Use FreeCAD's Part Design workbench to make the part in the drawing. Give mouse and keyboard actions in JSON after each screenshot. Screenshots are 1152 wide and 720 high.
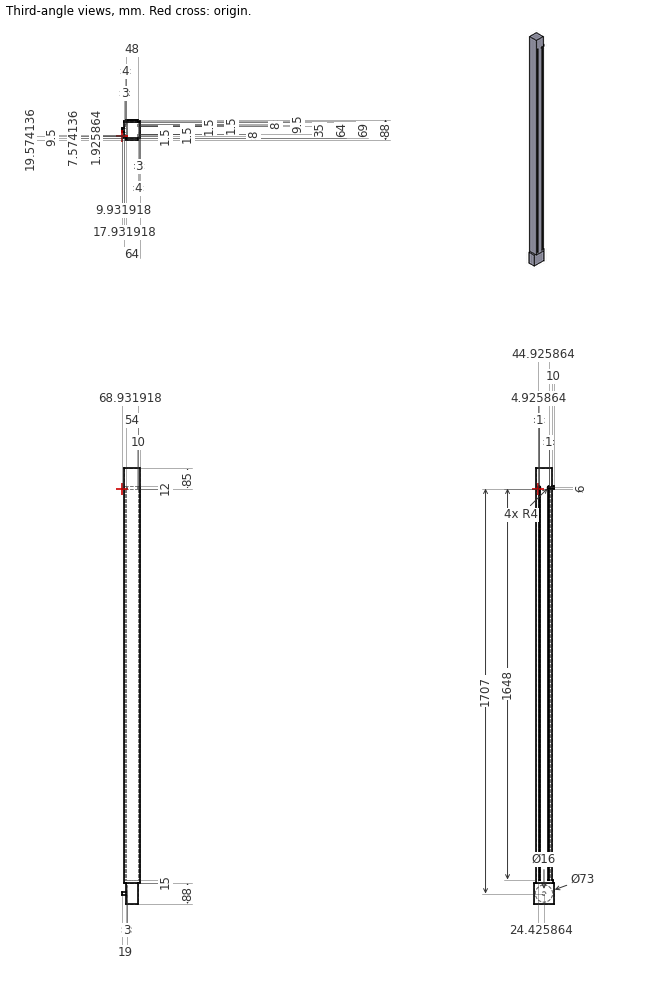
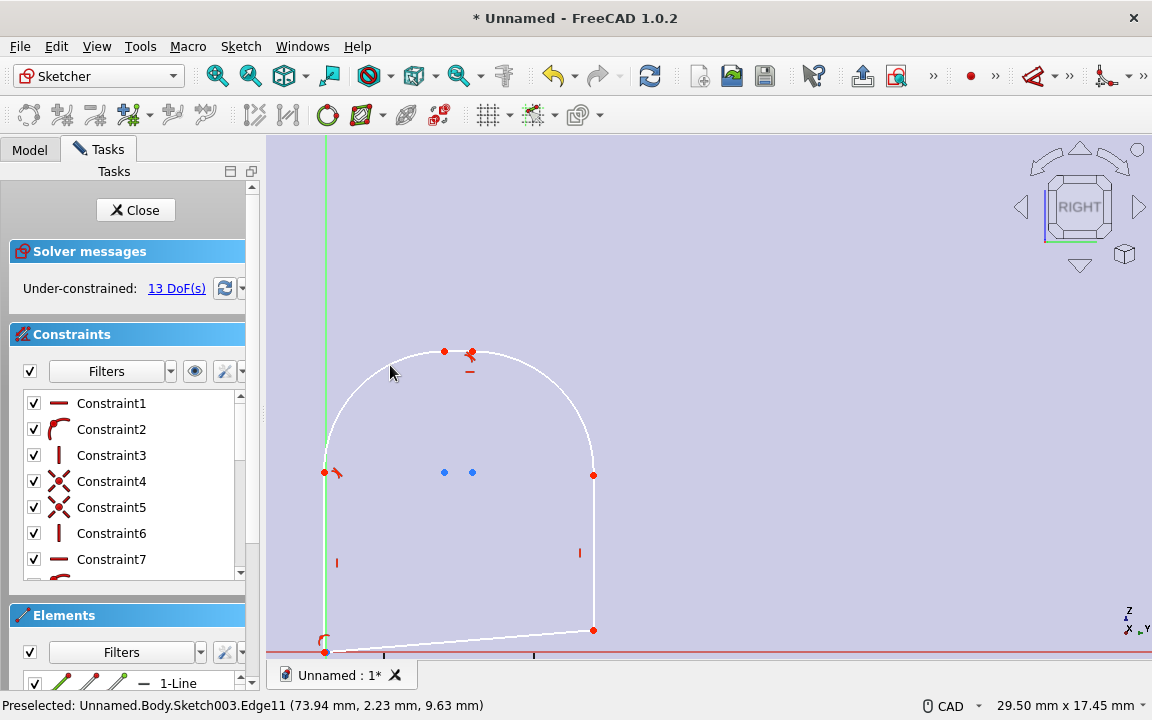
{"action": "left_click", "coordinate": [594, 584]}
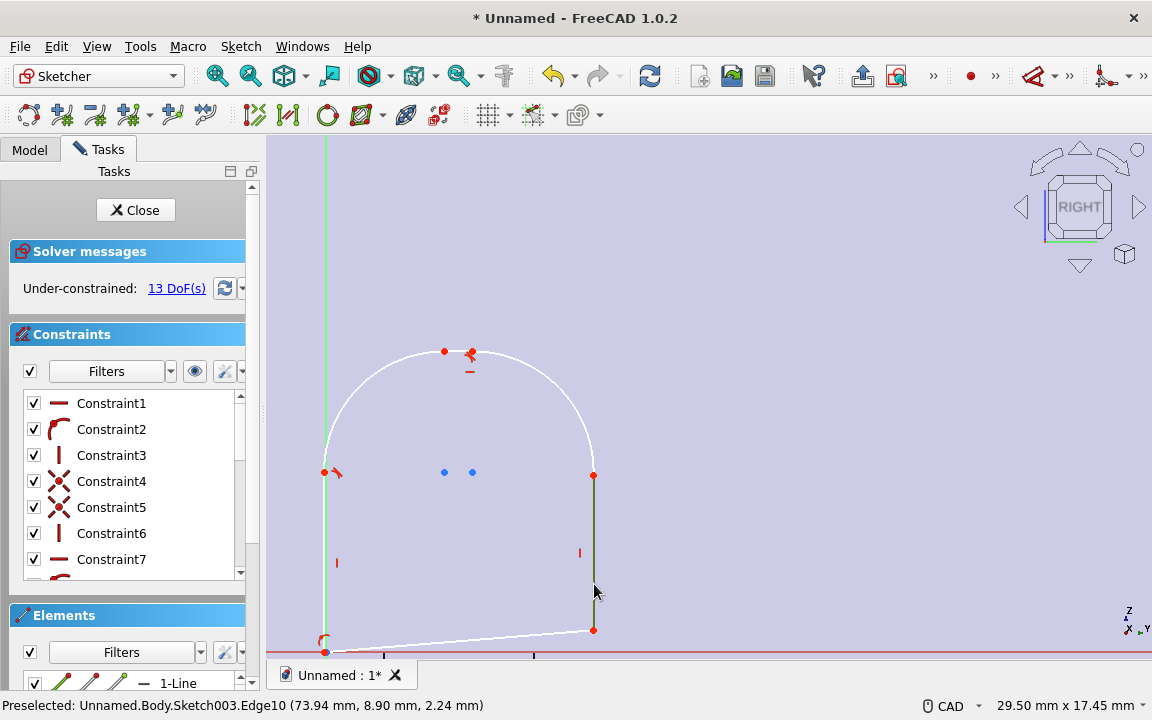
{"action": "left_click", "coordinate": [581, 419]}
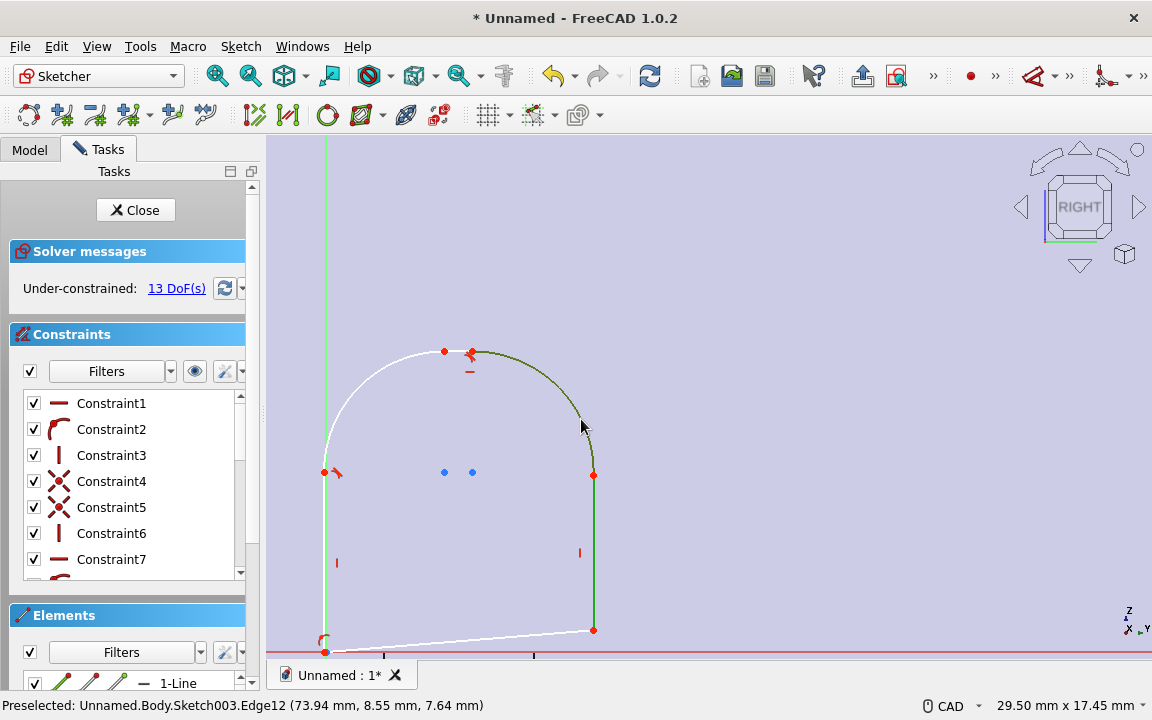
{"action": "key", "text": "t"}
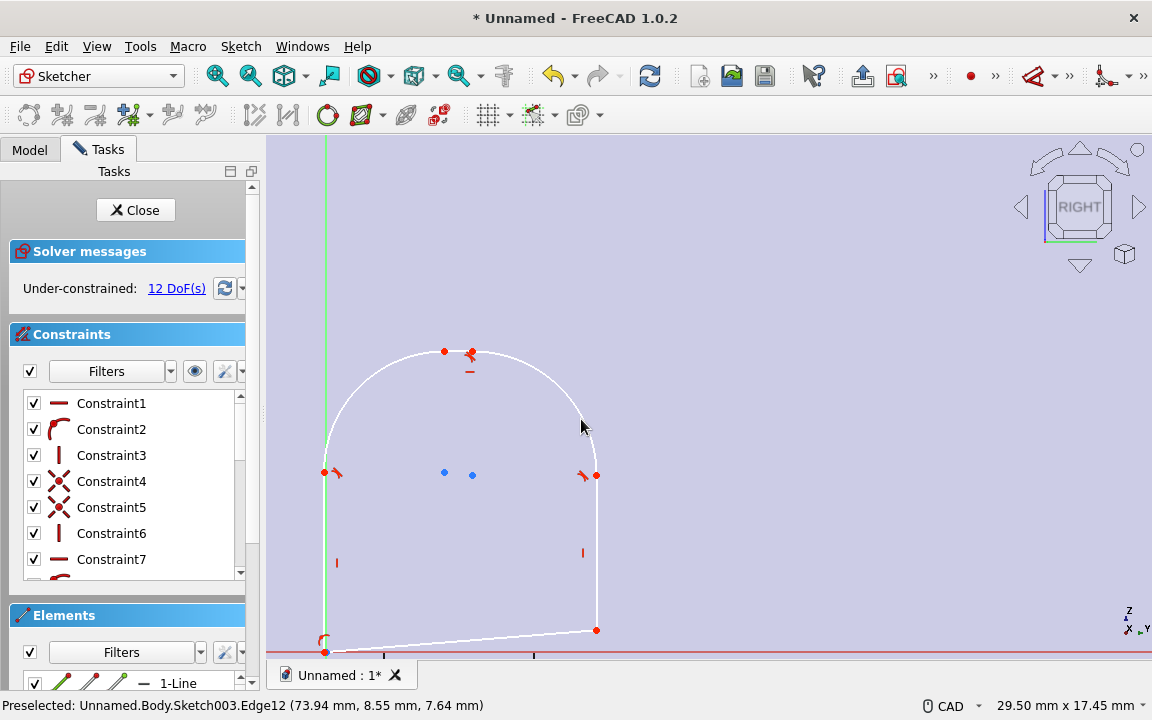
{"action": "scroll", "coordinate": [460, 352], "scroll_direction": "down", "scroll_amount": 6}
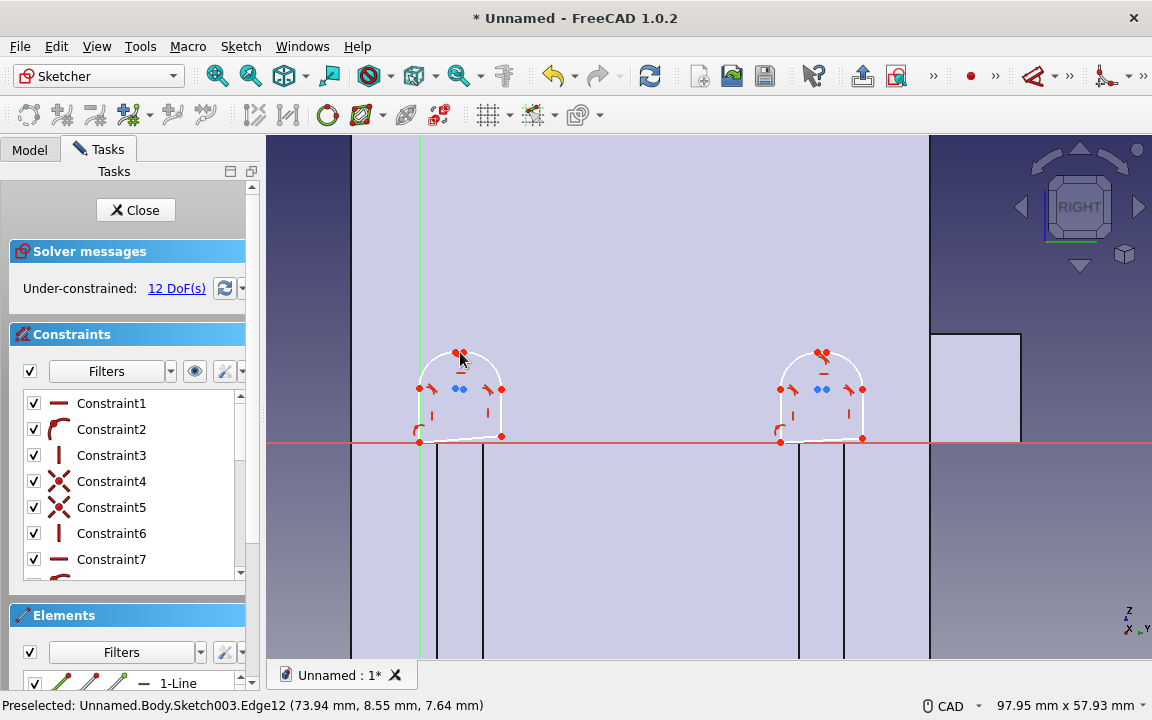
{"action": "scroll", "coordinate": [838, 440], "scroll_direction": "up", "scroll_amount": 8}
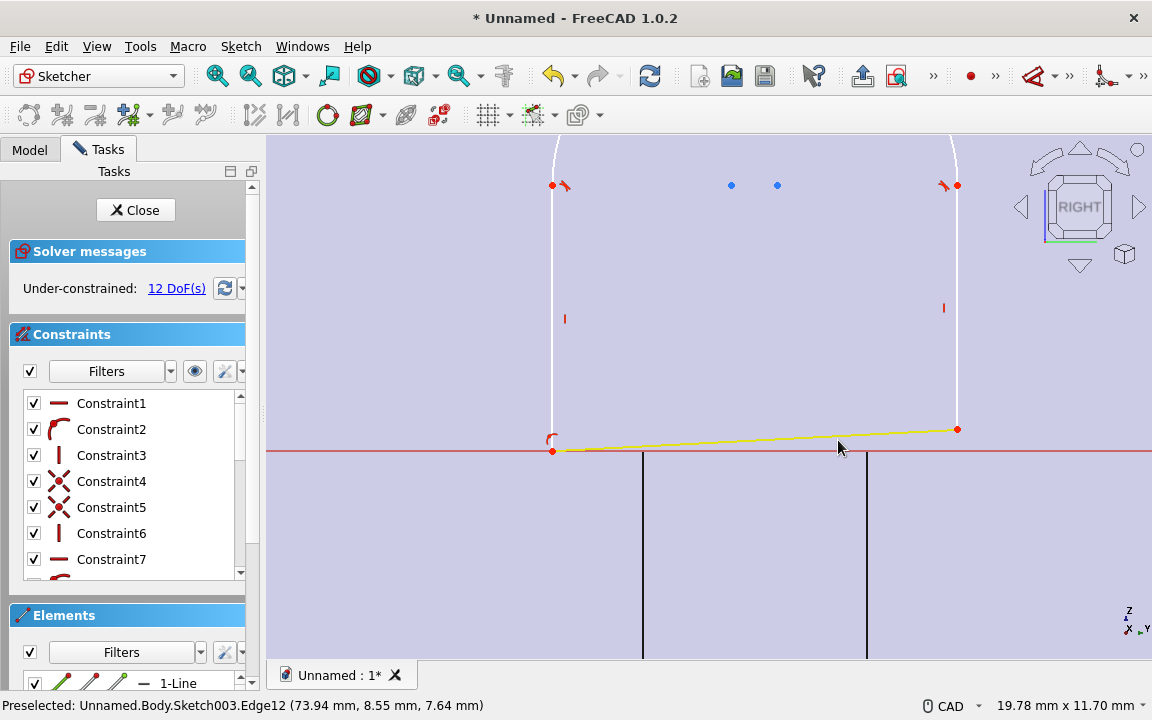
{"action": "left_click", "coordinate": [836, 436]}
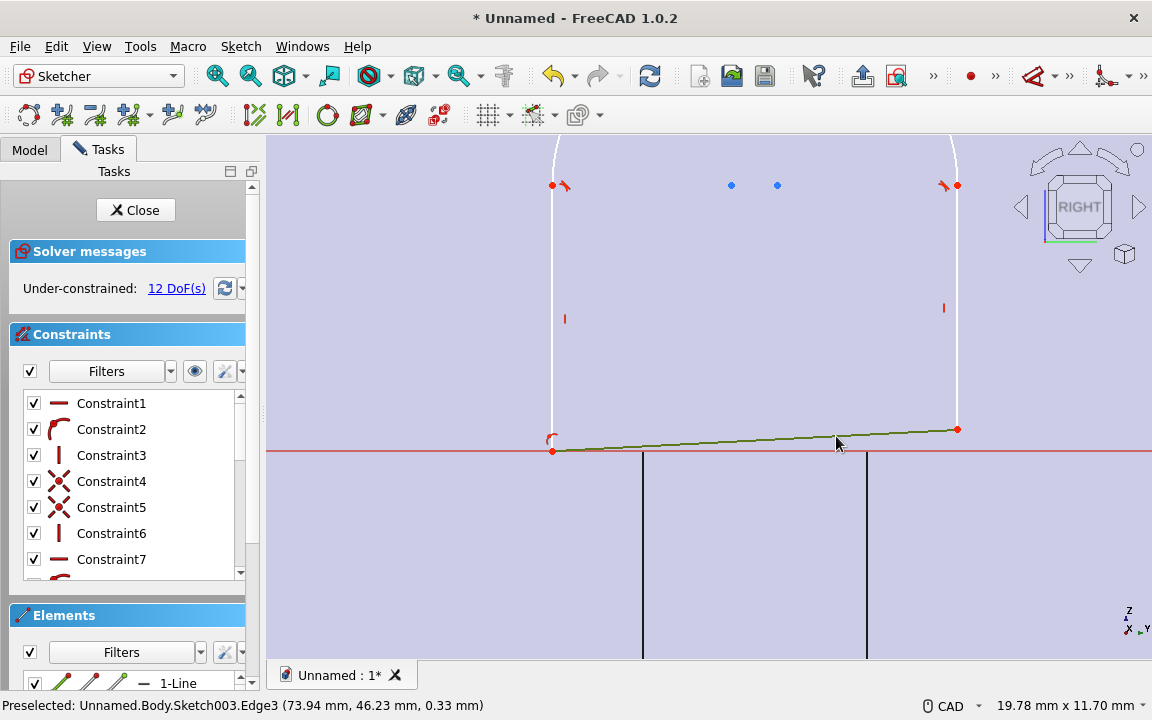
{"action": "key", "text": "h"}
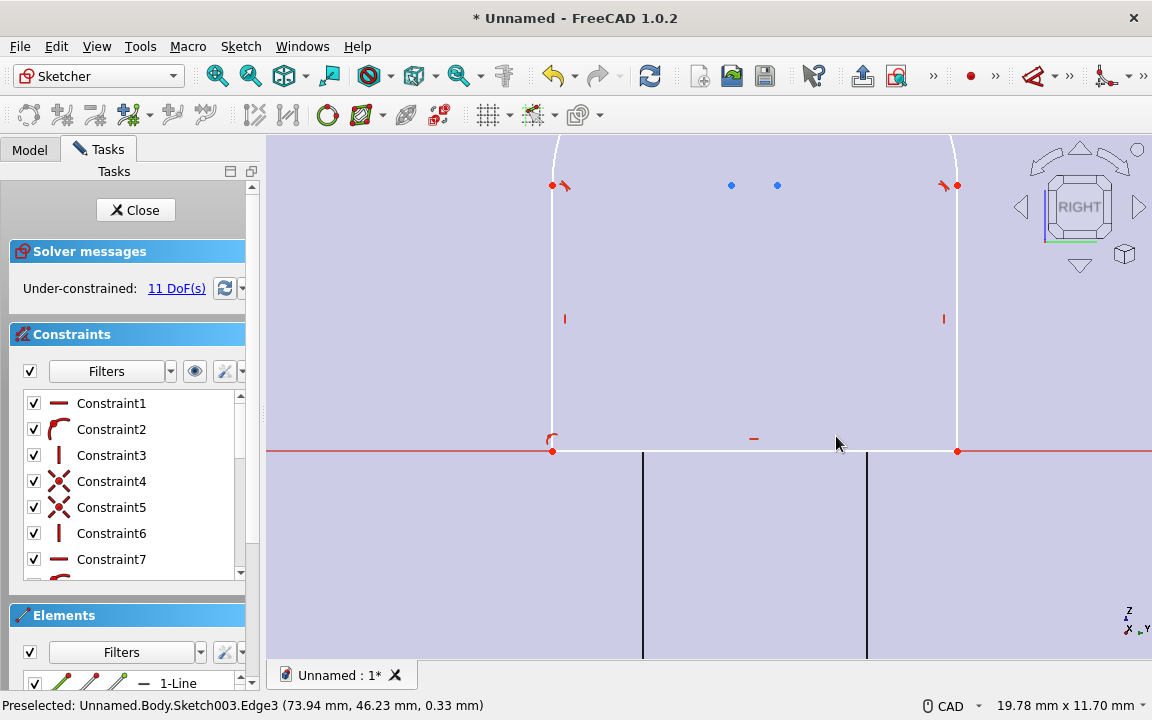
{"action": "scroll", "coordinate": [838, 440], "scroll_direction": "down", "scroll_amount": 8}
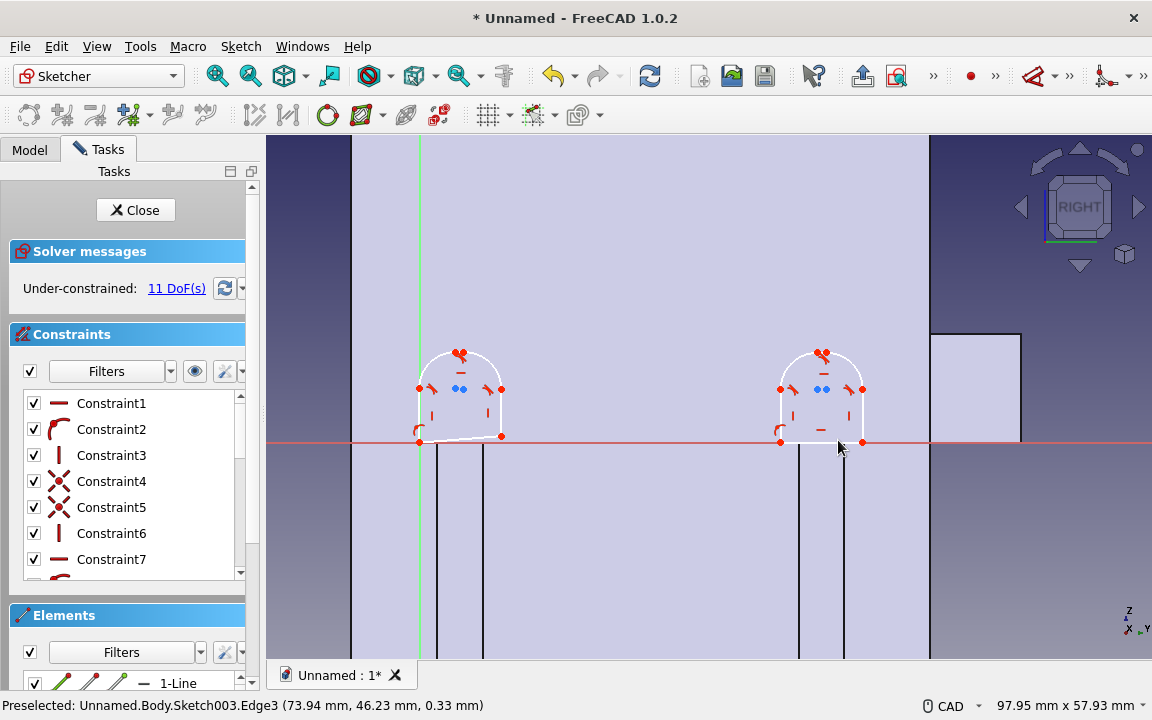
{"action": "scroll", "coordinate": [444, 441], "scroll_direction": "up", "scroll_amount": 10}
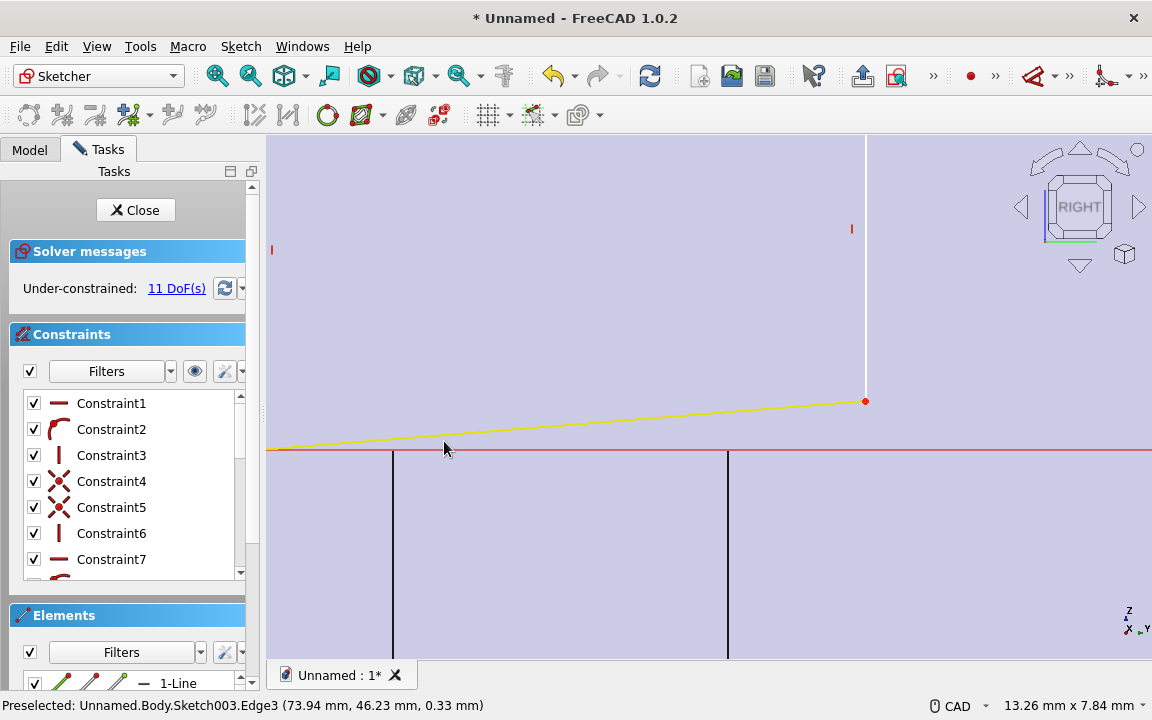
{"action": "left_click", "coordinate": [441, 435]}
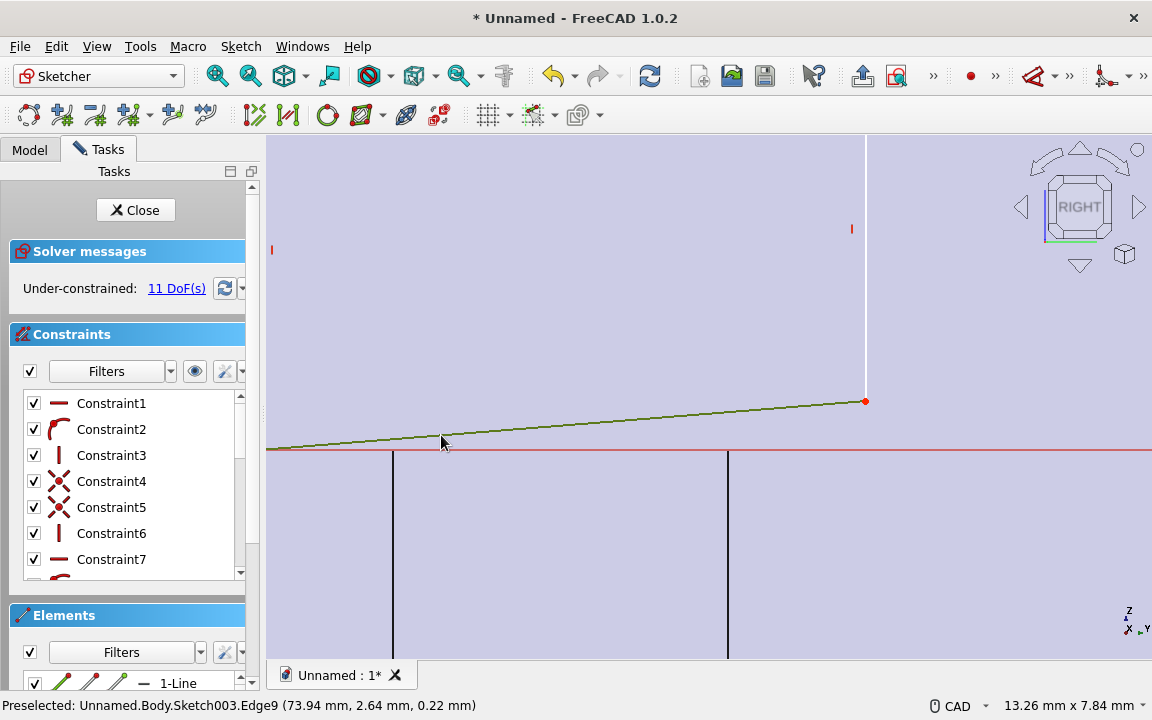
{"action": "key", "text": "h"}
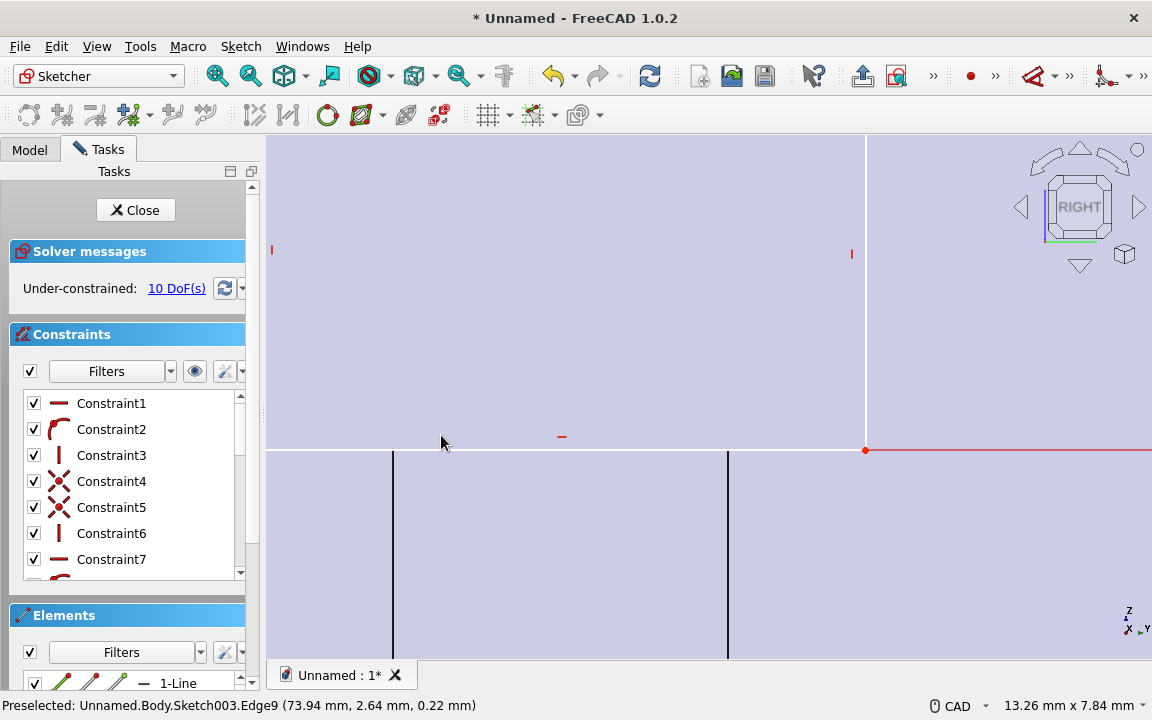
{"action": "scroll", "coordinate": [444, 441], "scroll_direction": "down", "scroll_amount": 10}